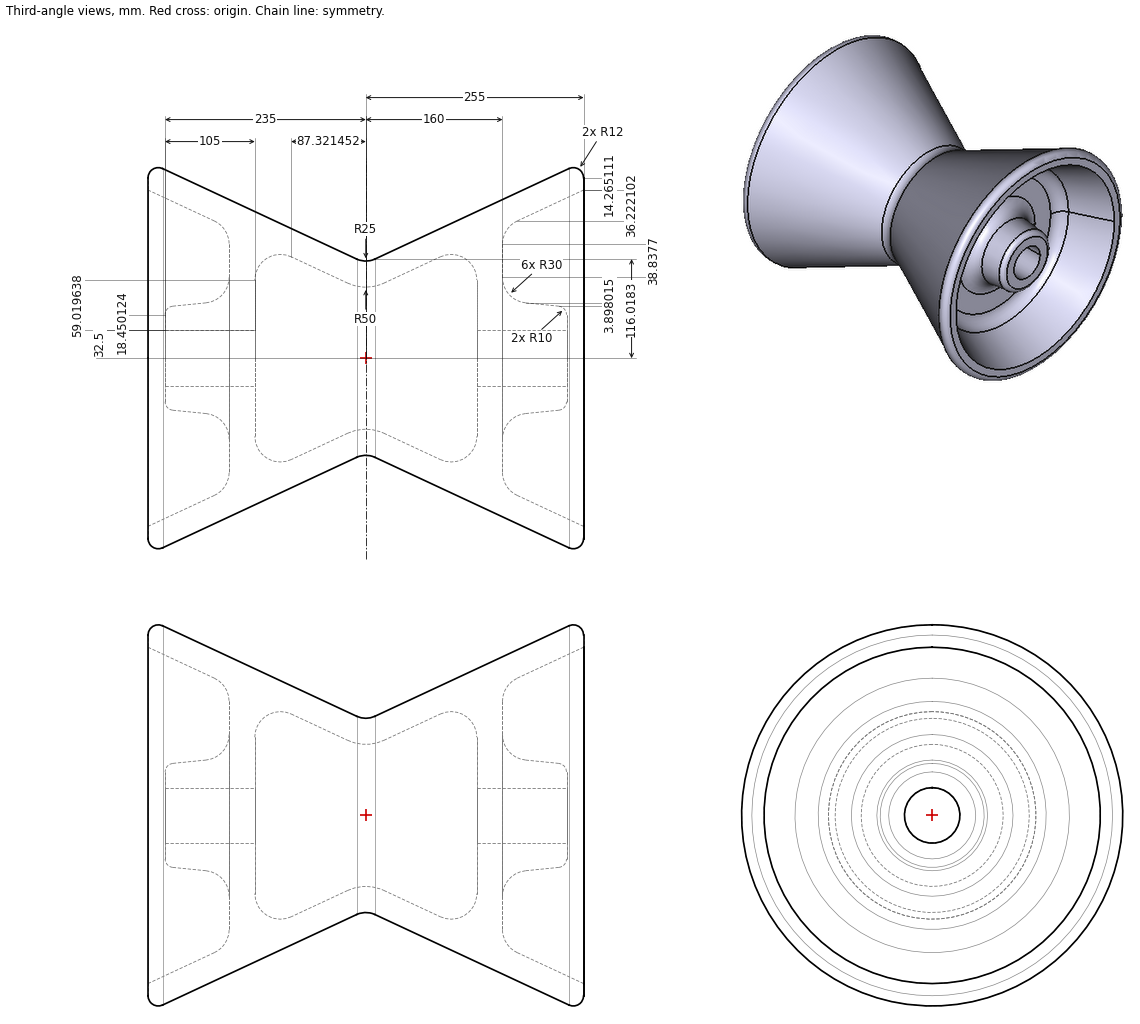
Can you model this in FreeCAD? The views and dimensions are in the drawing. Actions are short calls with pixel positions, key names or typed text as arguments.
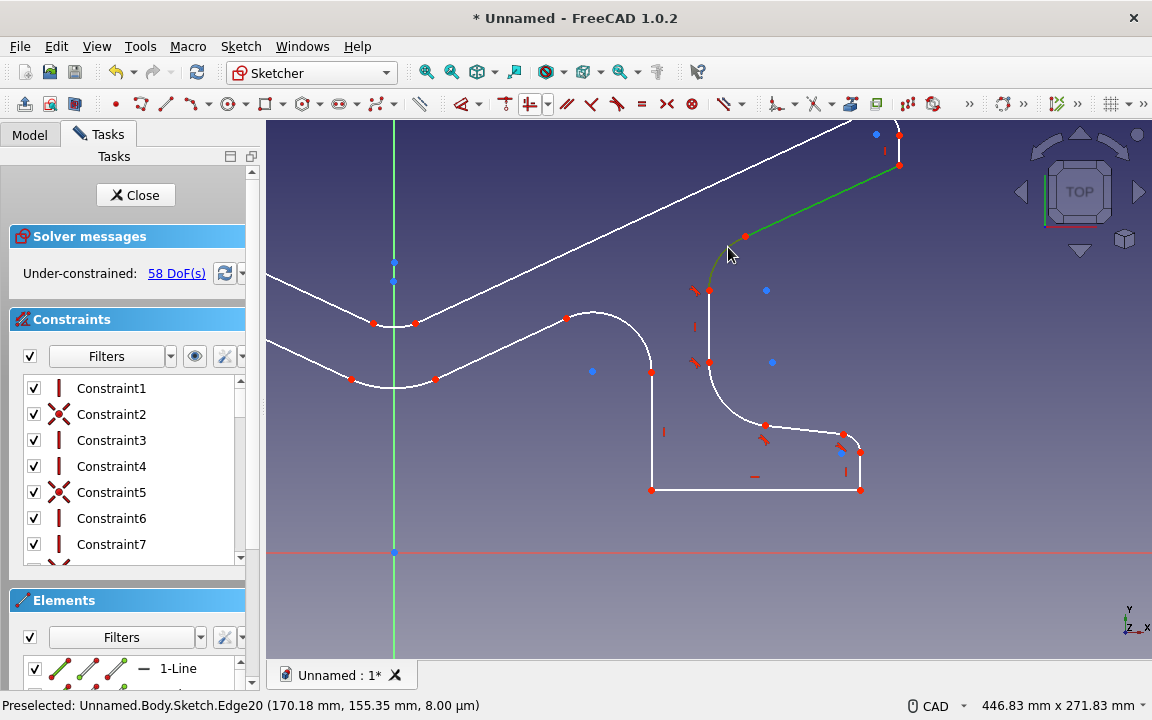
key(t)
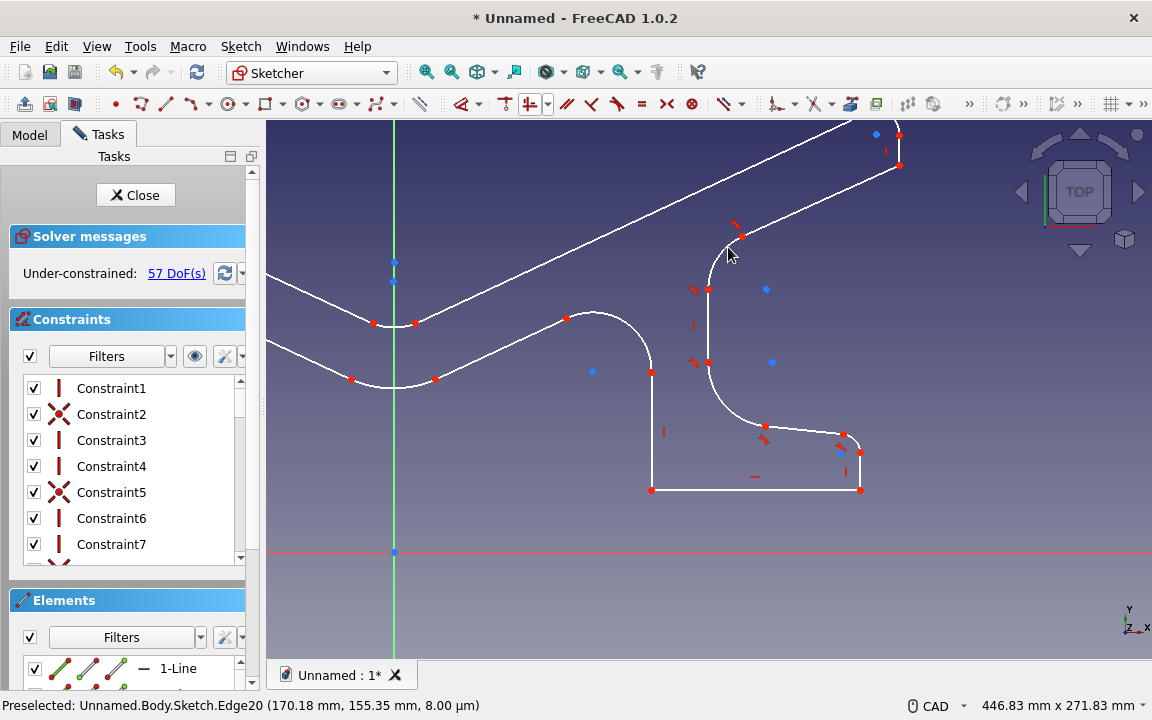
click(899, 154)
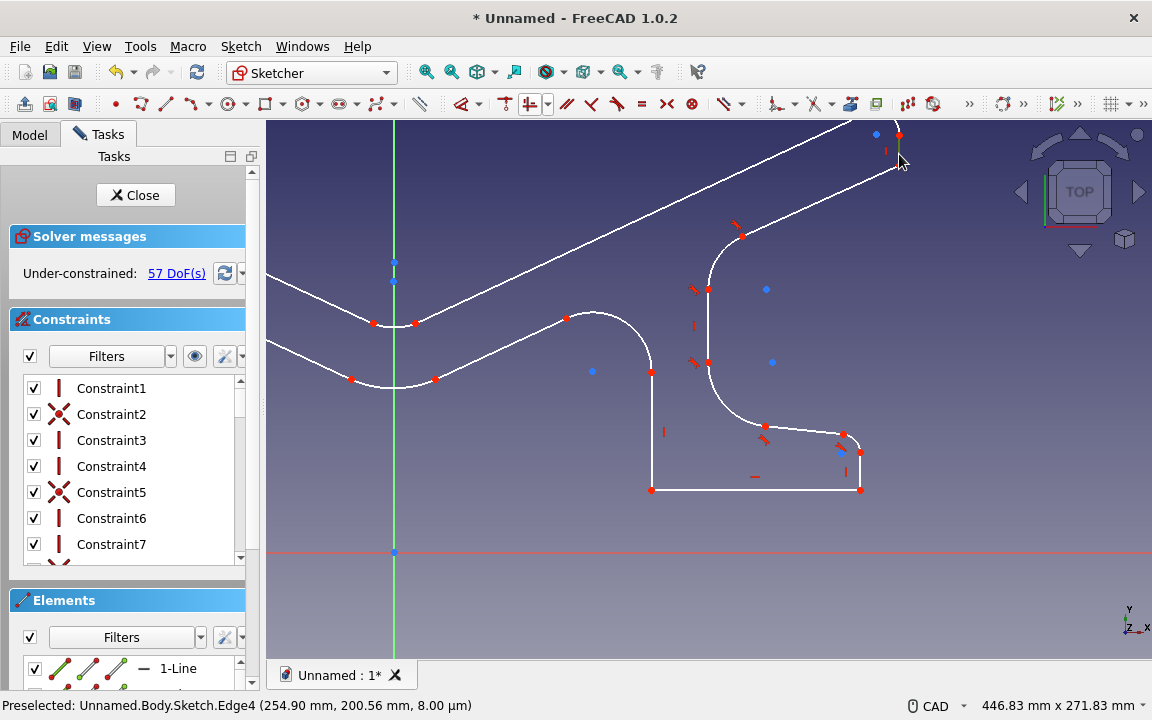
scroll(842, 436, down, 4)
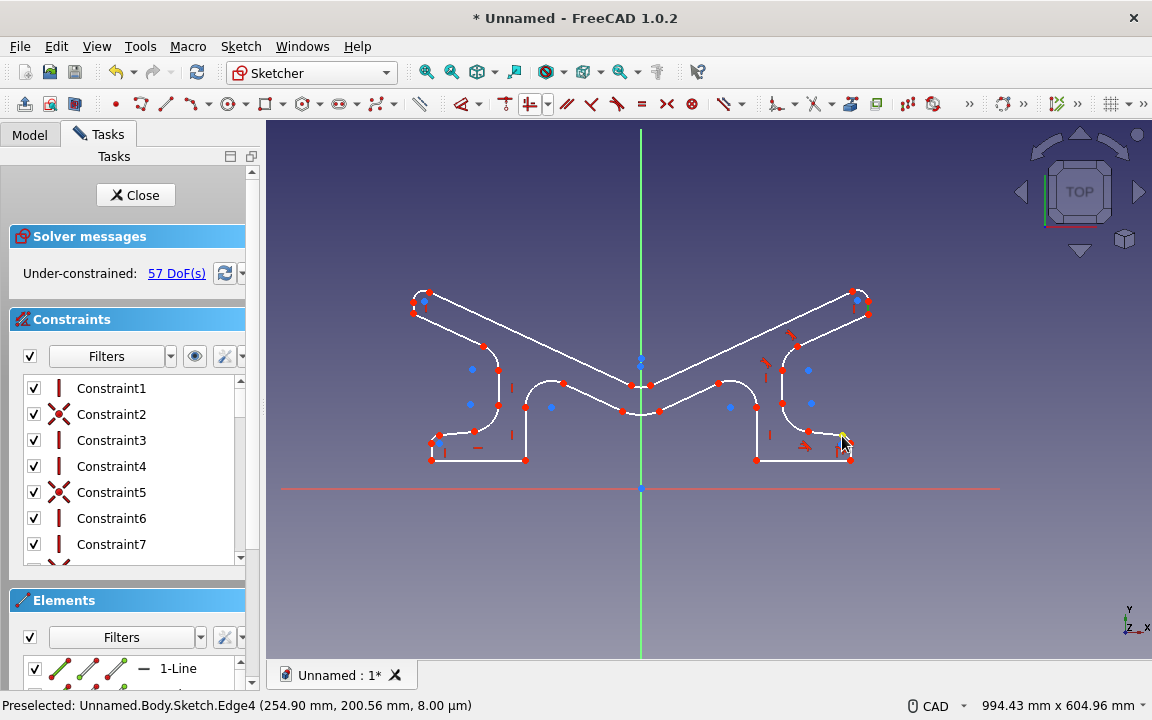
scroll(867, 295, up, 4)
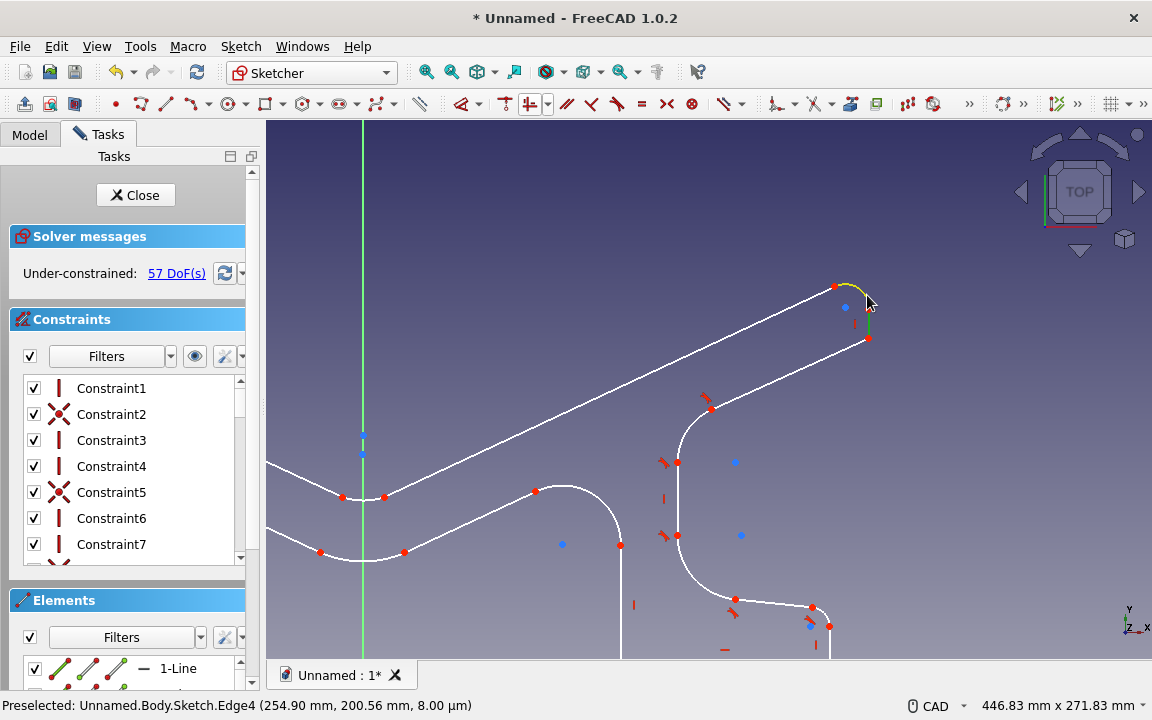
click(865, 295)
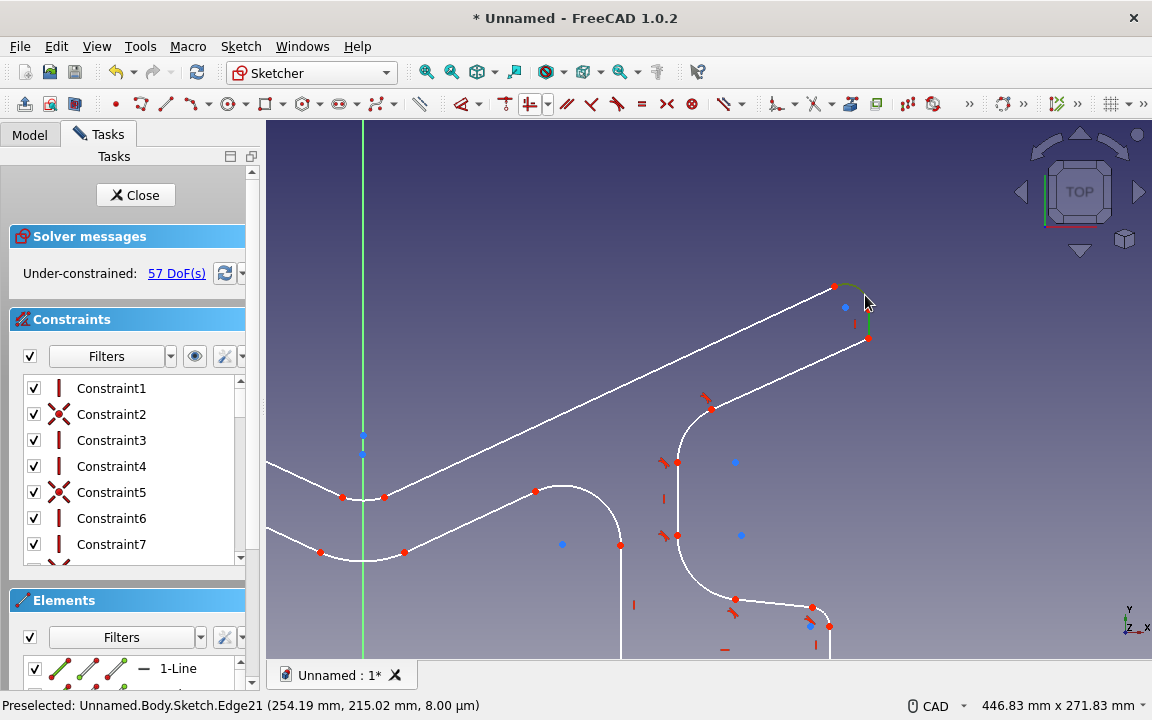
click(617, 104)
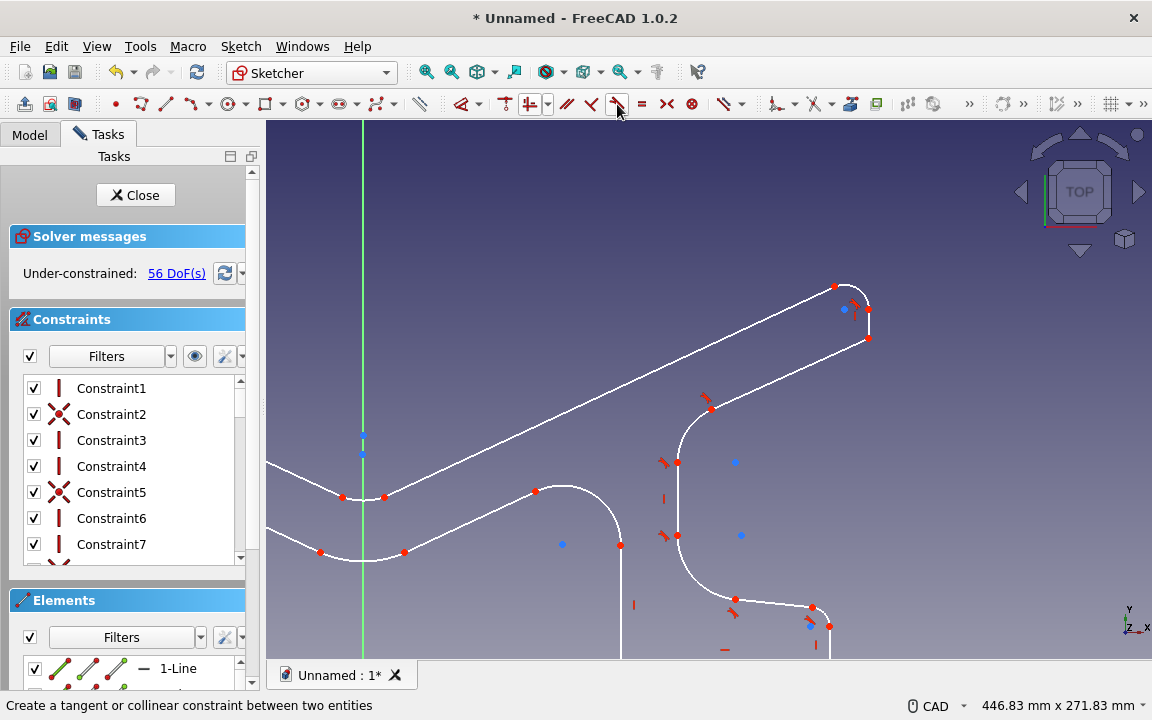
click(700, 350)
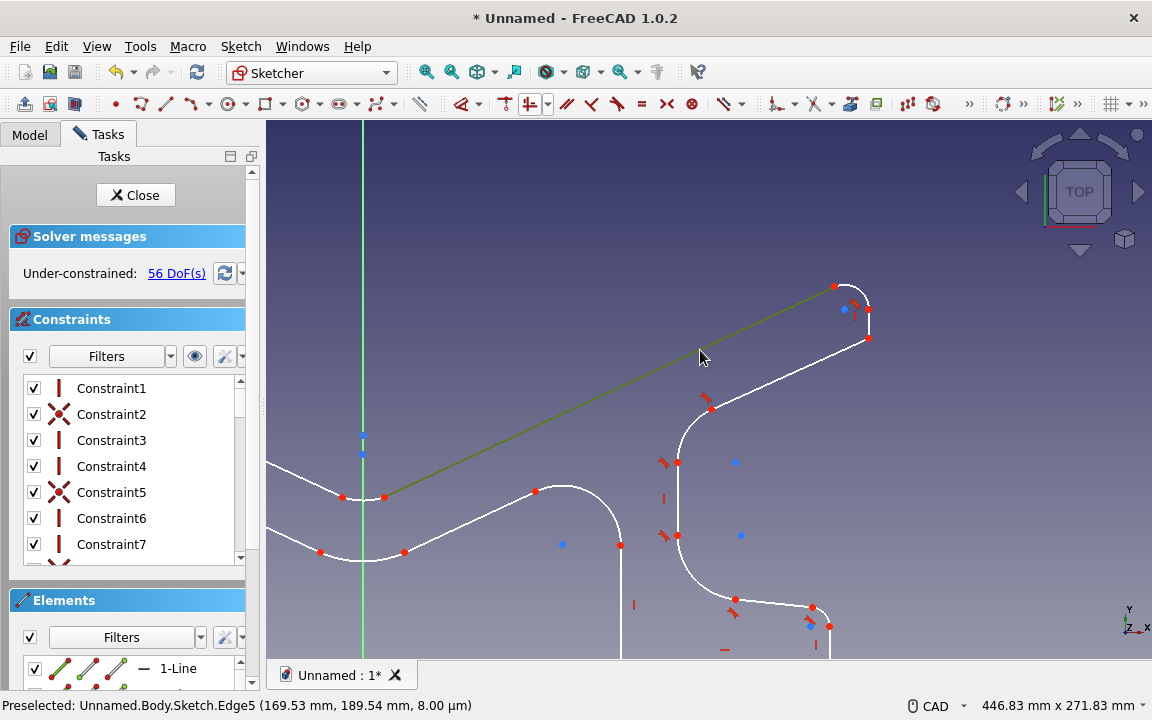
click(865, 296)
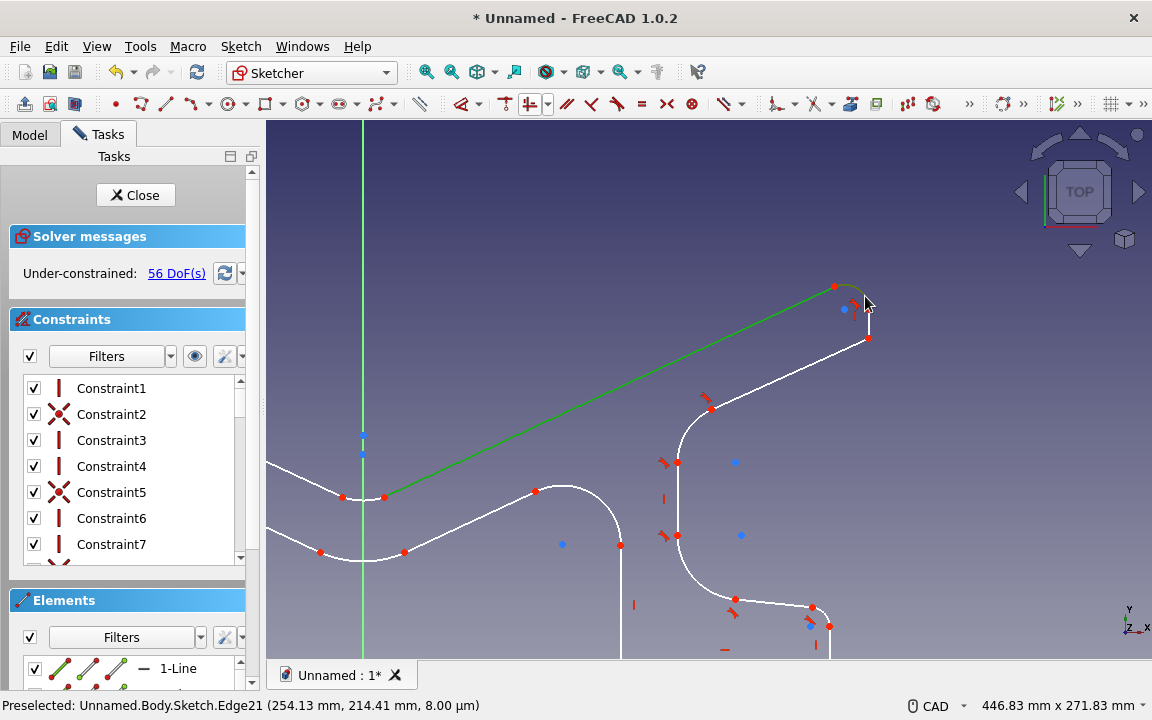
click(617, 104)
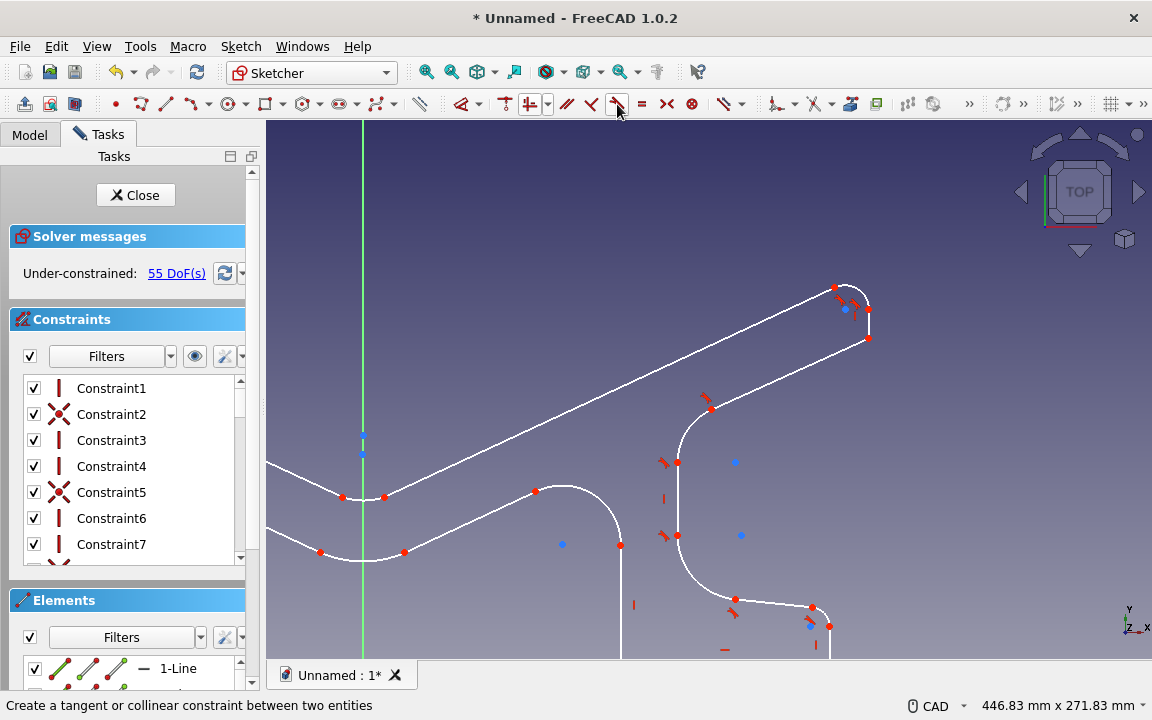
click(700, 350)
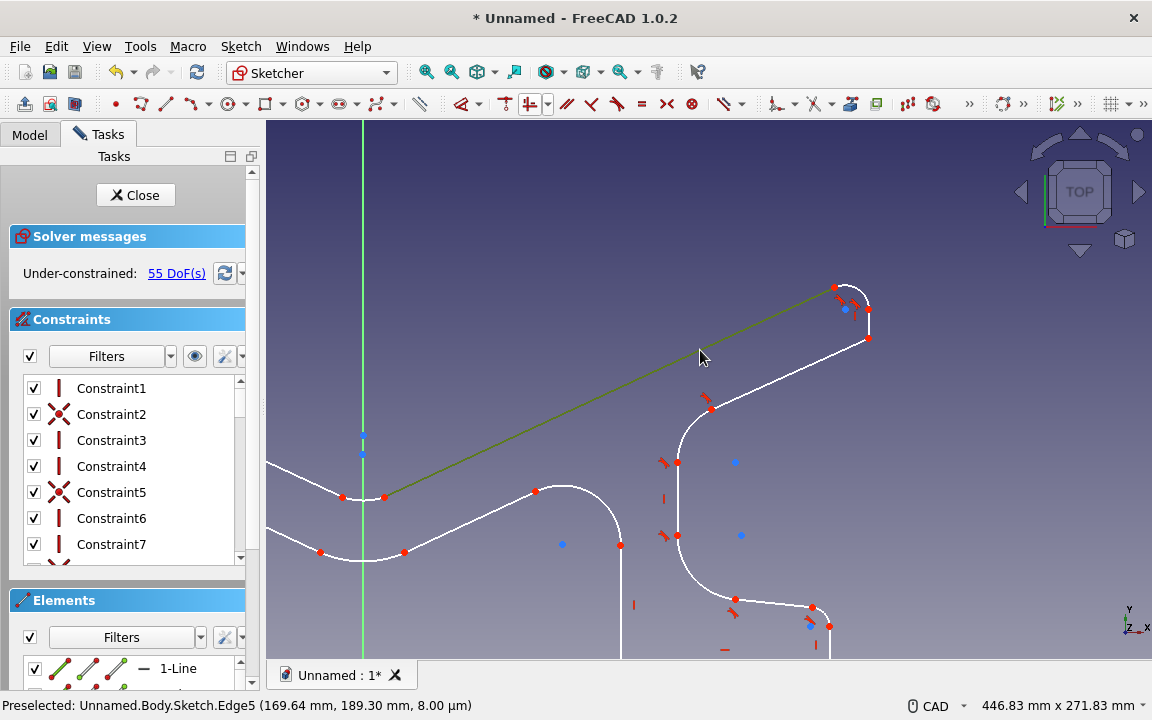
click(364, 501)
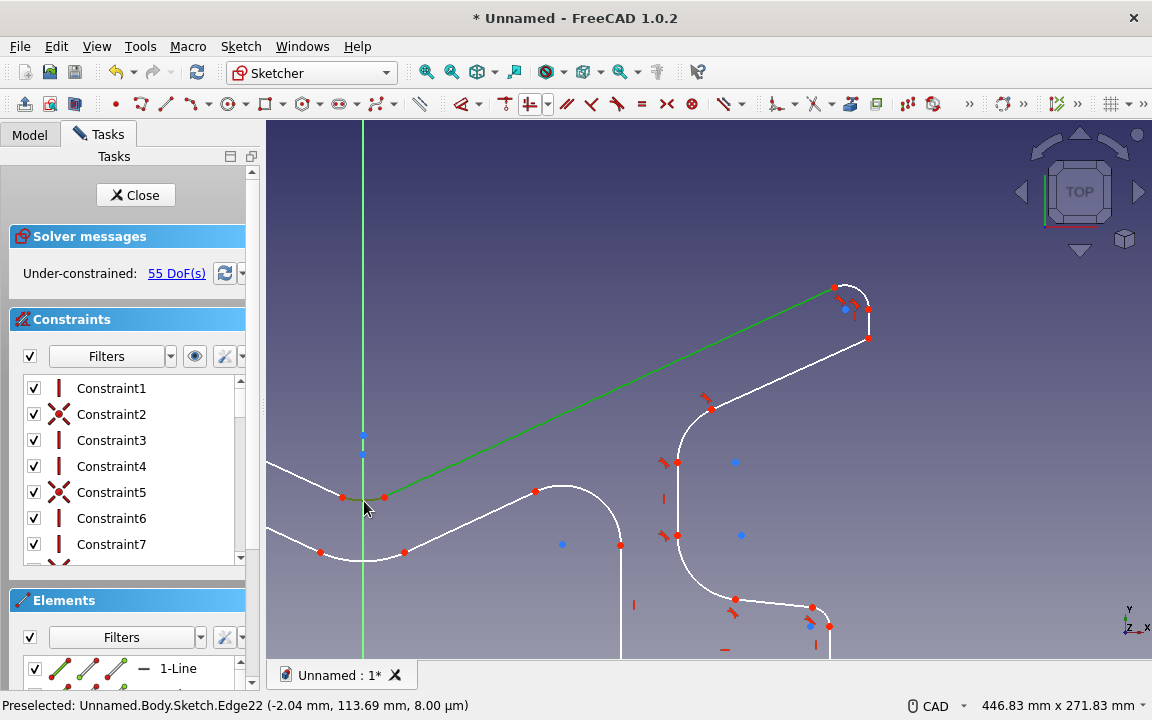
click(617, 104)